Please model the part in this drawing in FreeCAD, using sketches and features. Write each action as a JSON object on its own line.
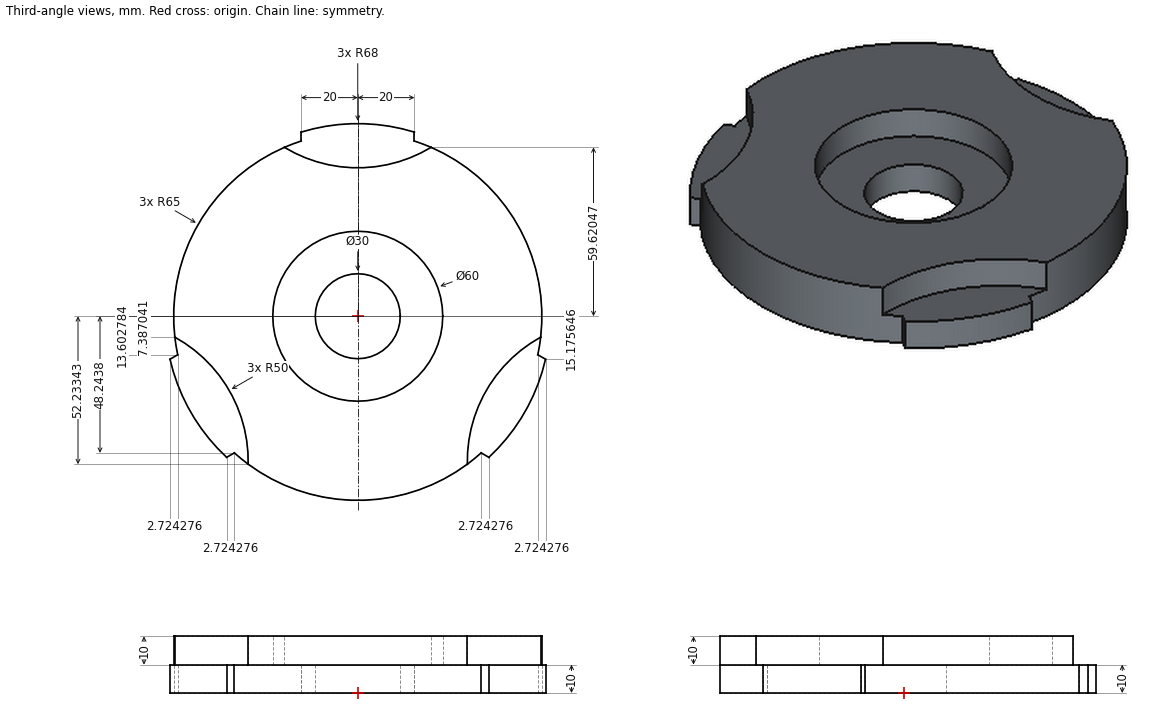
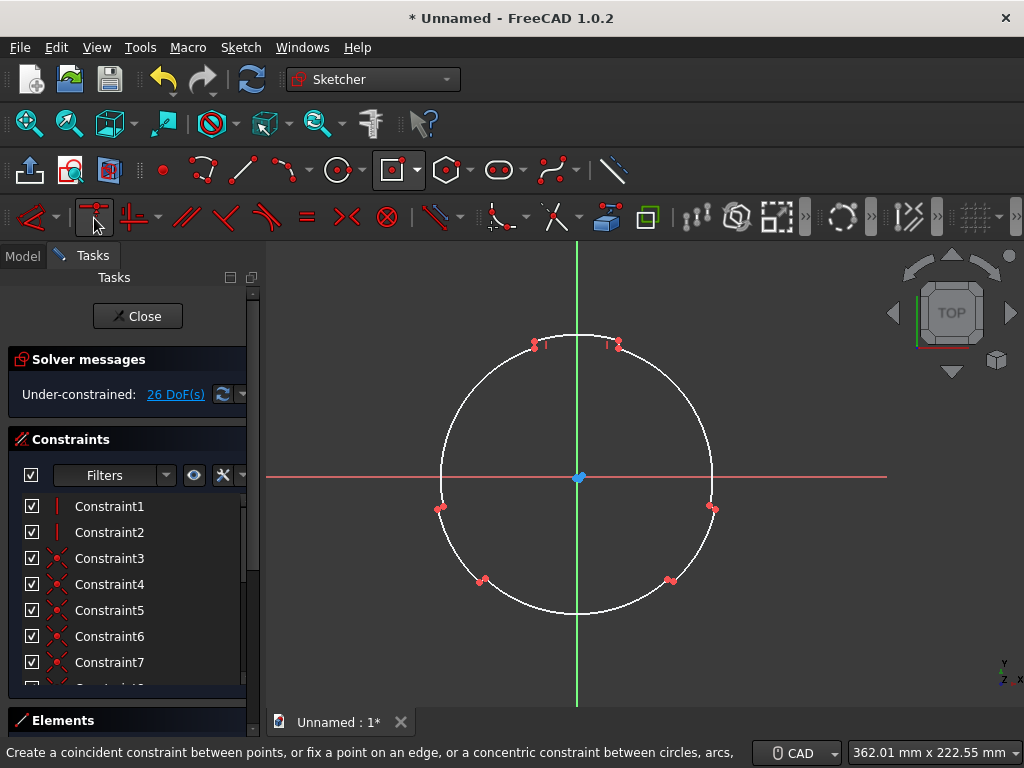
{"action": "left_click", "coordinate": [594, 335]}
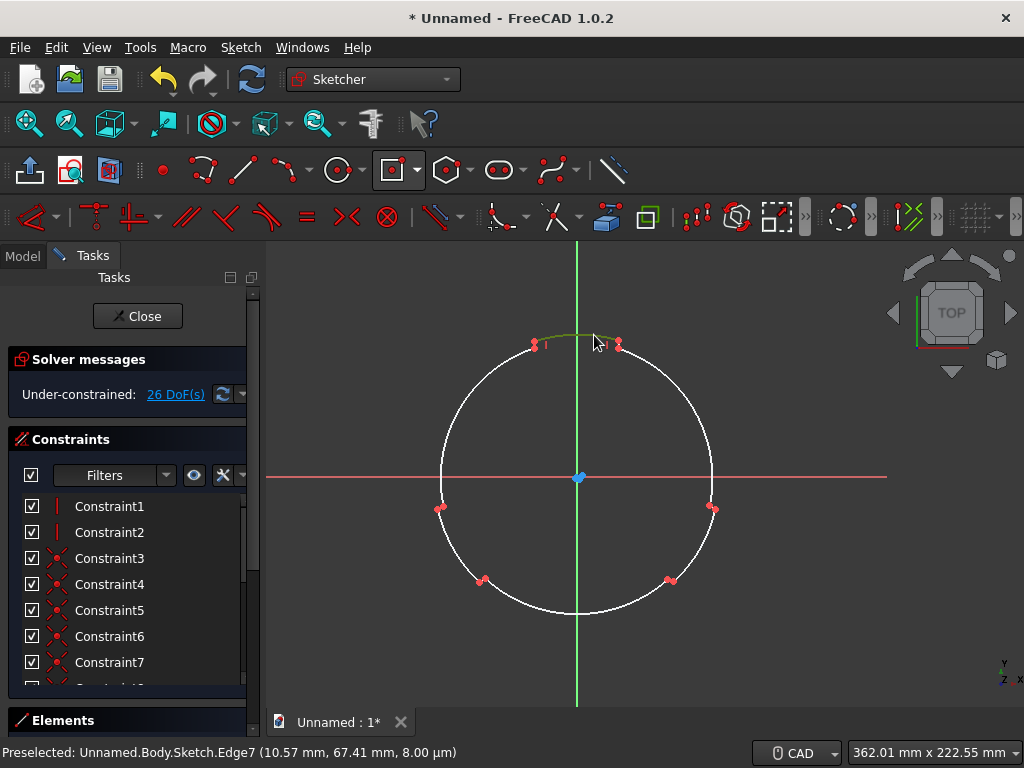
{"action": "left_click", "coordinate": [446, 534]}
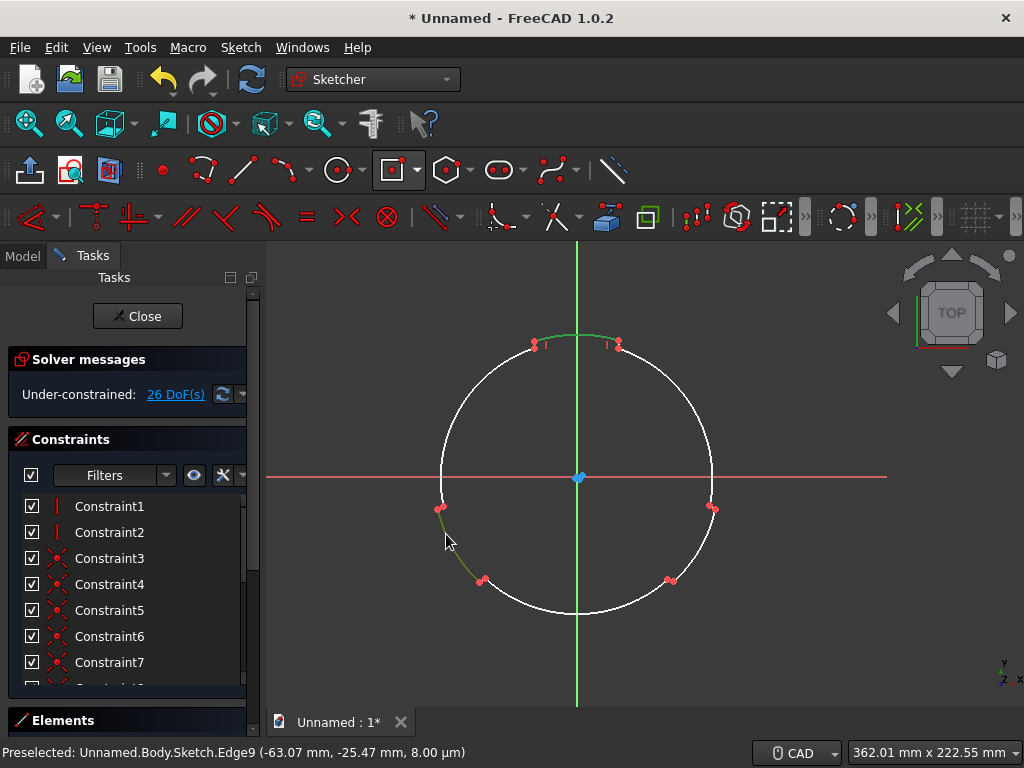
{"action": "left_click", "coordinate": [94, 218]}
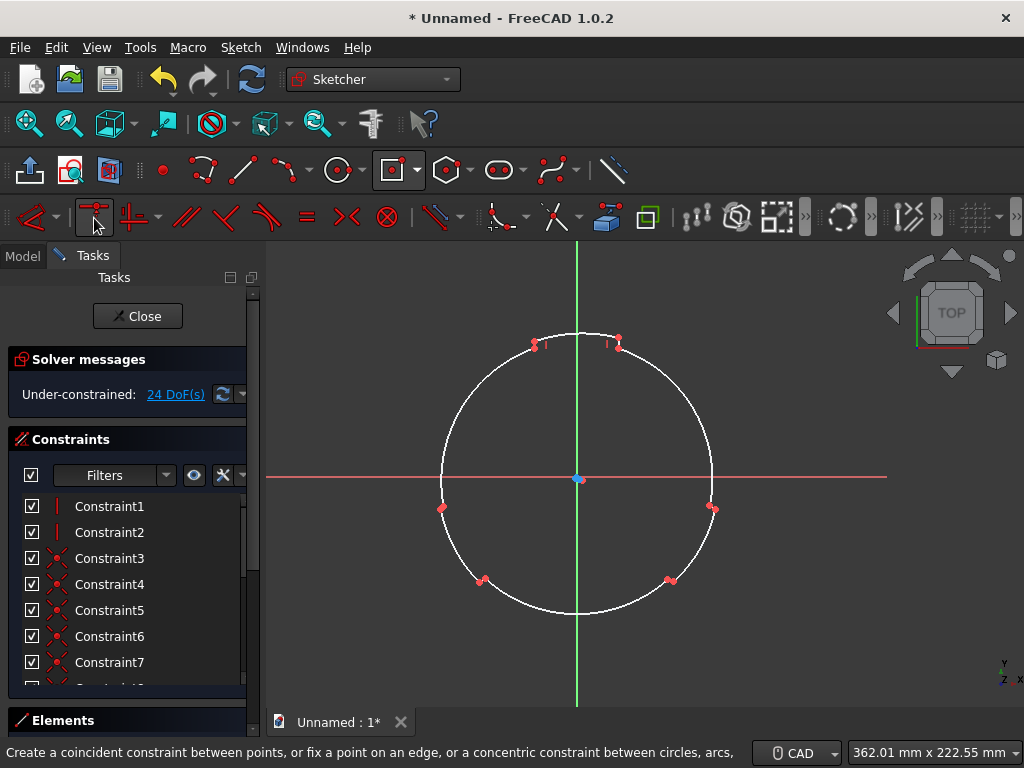
{"action": "left_click", "coordinate": [593, 334]}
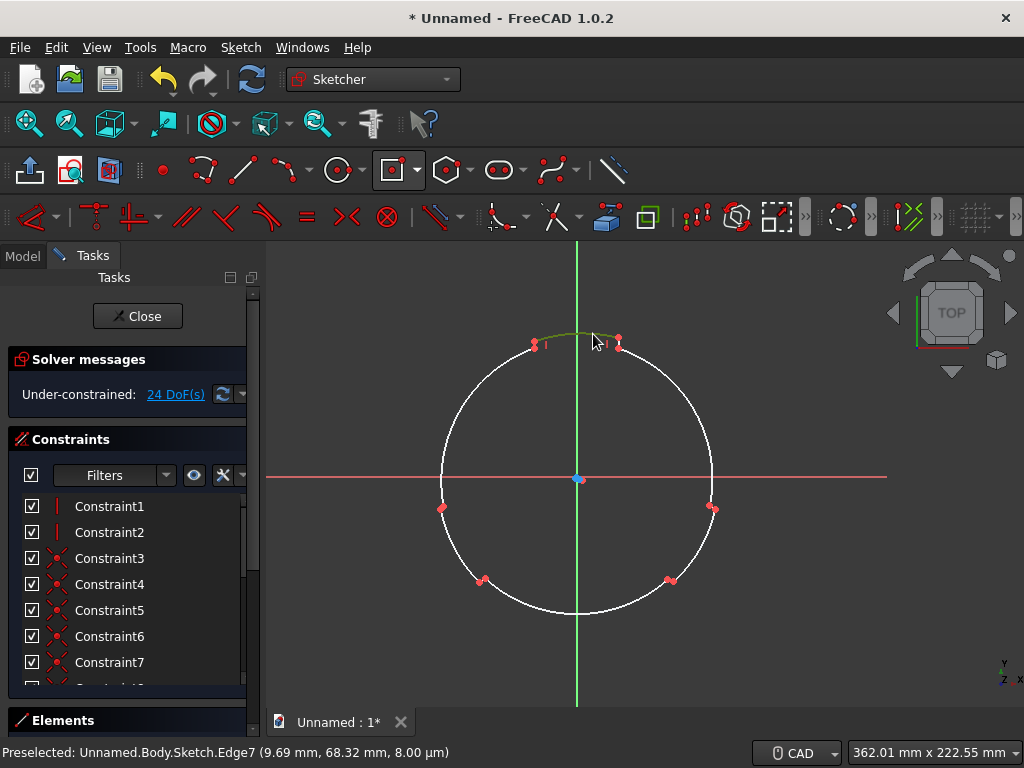
{"action": "left_click", "coordinate": [537, 608]}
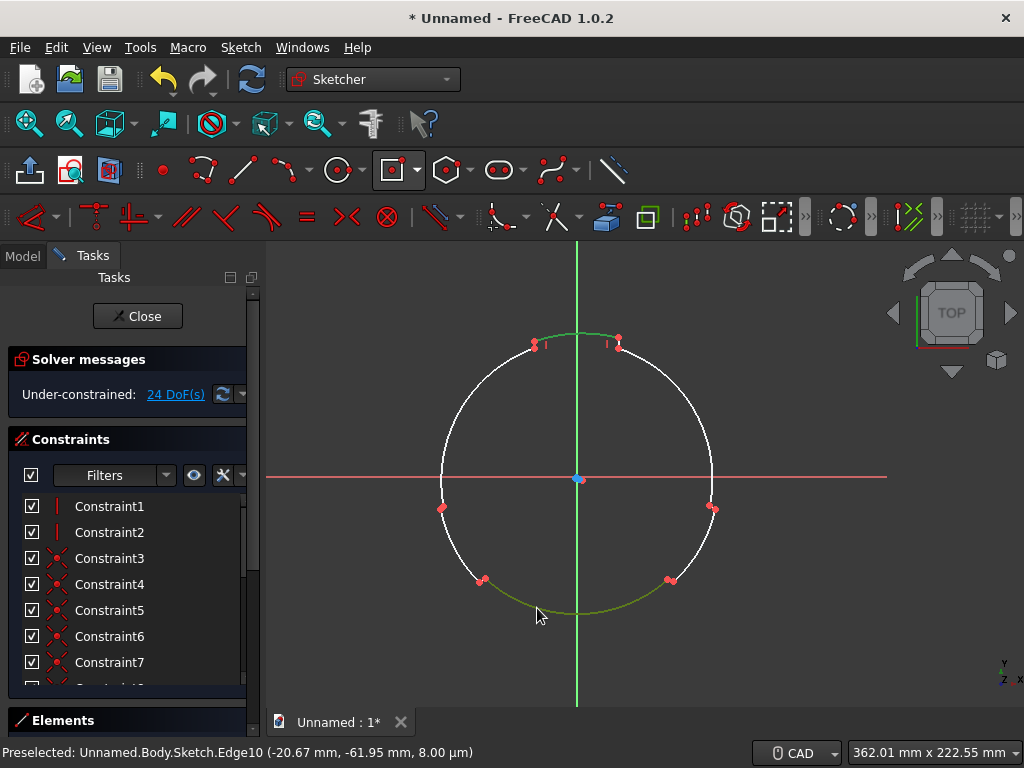
{"action": "left_click", "coordinate": [94, 218]}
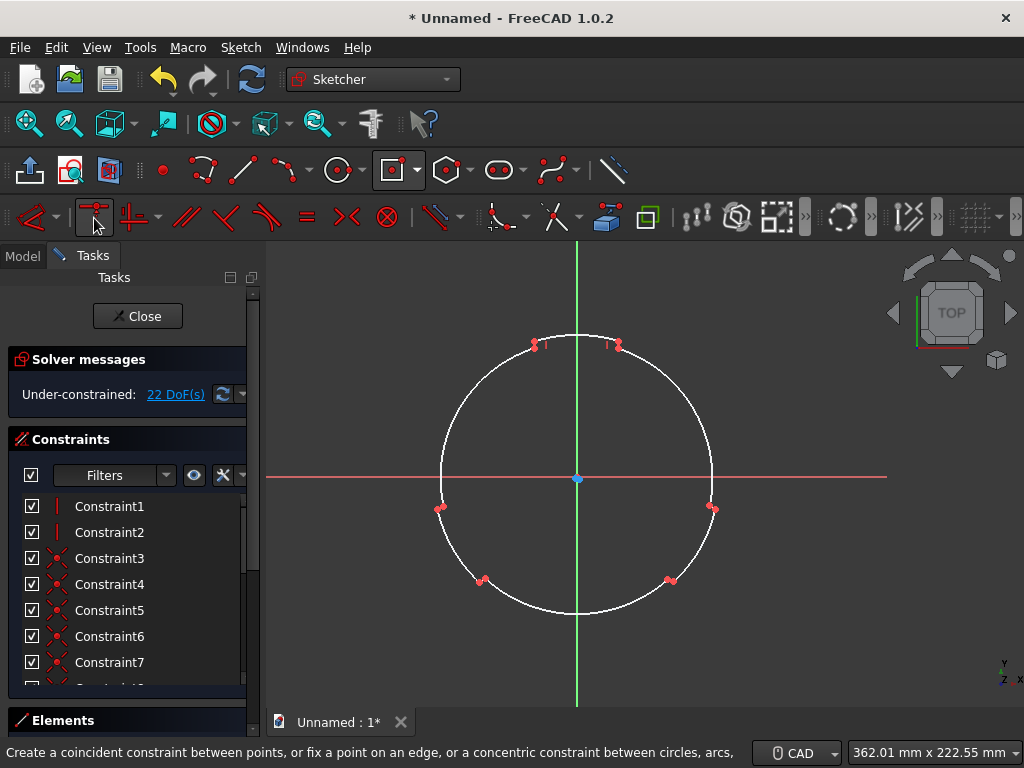
{"action": "left_click", "coordinate": [594, 336]}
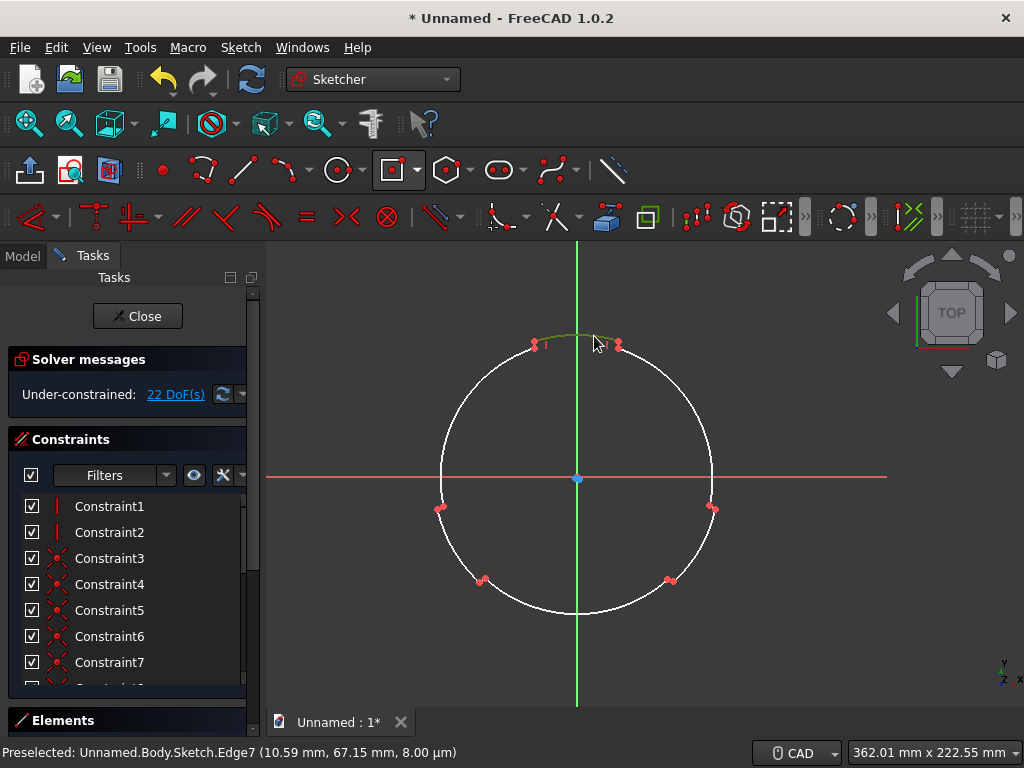
{"action": "left_click", "coordinate": [691, 563]}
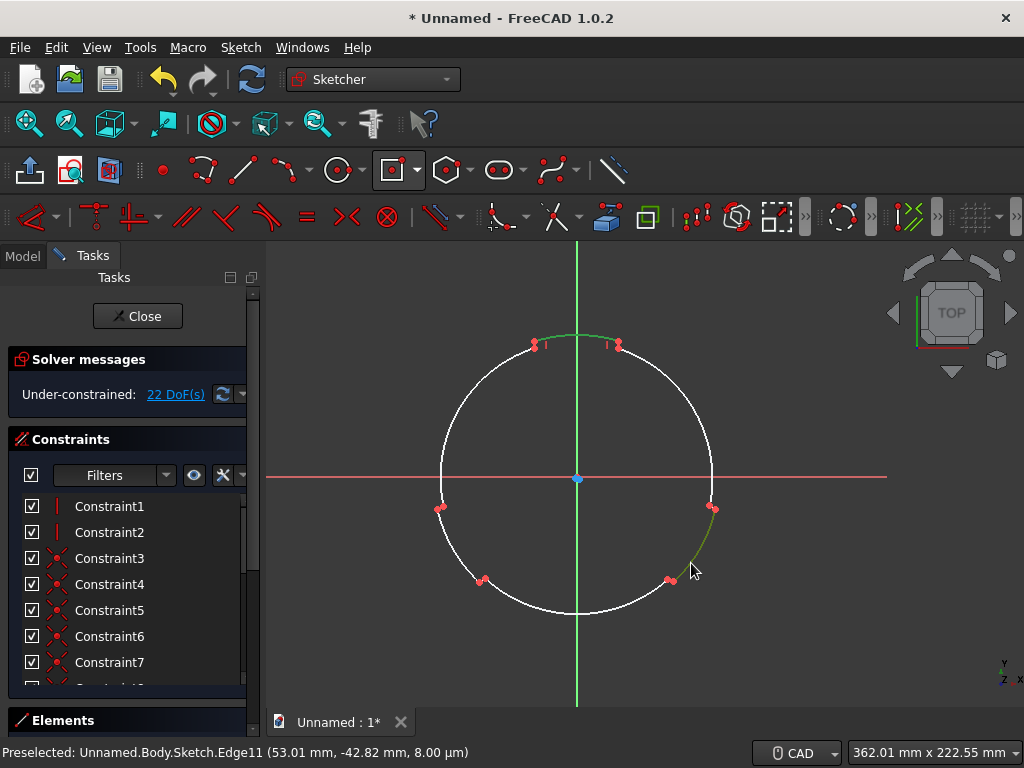
{"action": "key", "text": "c"}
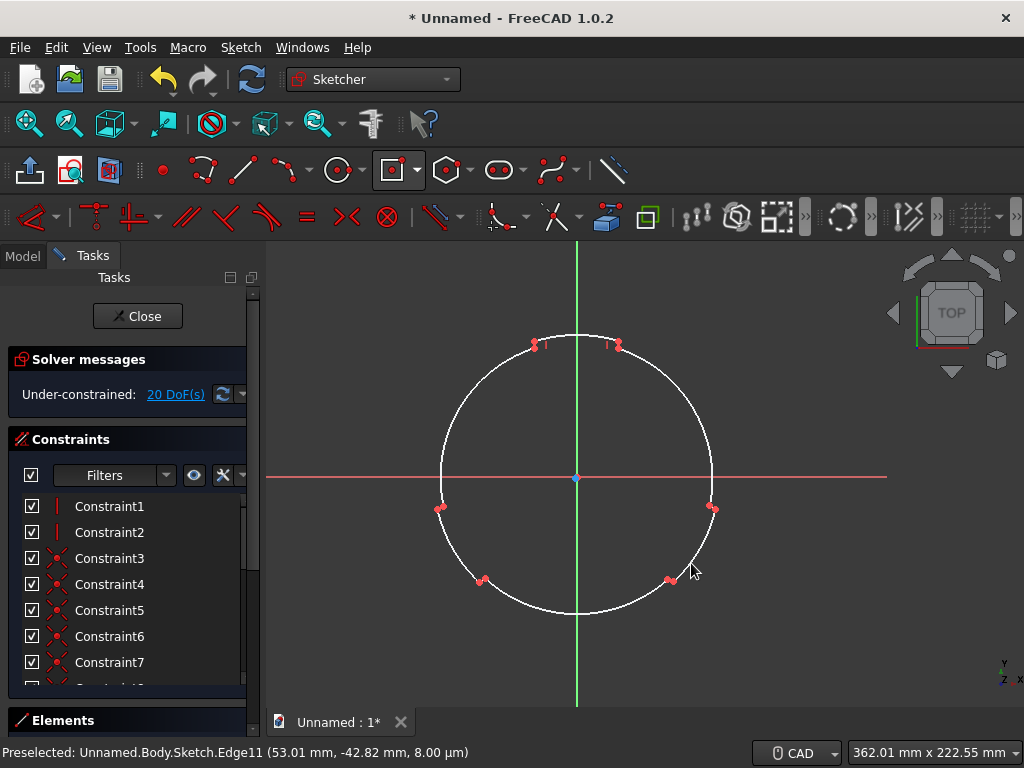
{"action": "left_click", "coordinate": [594, 336]}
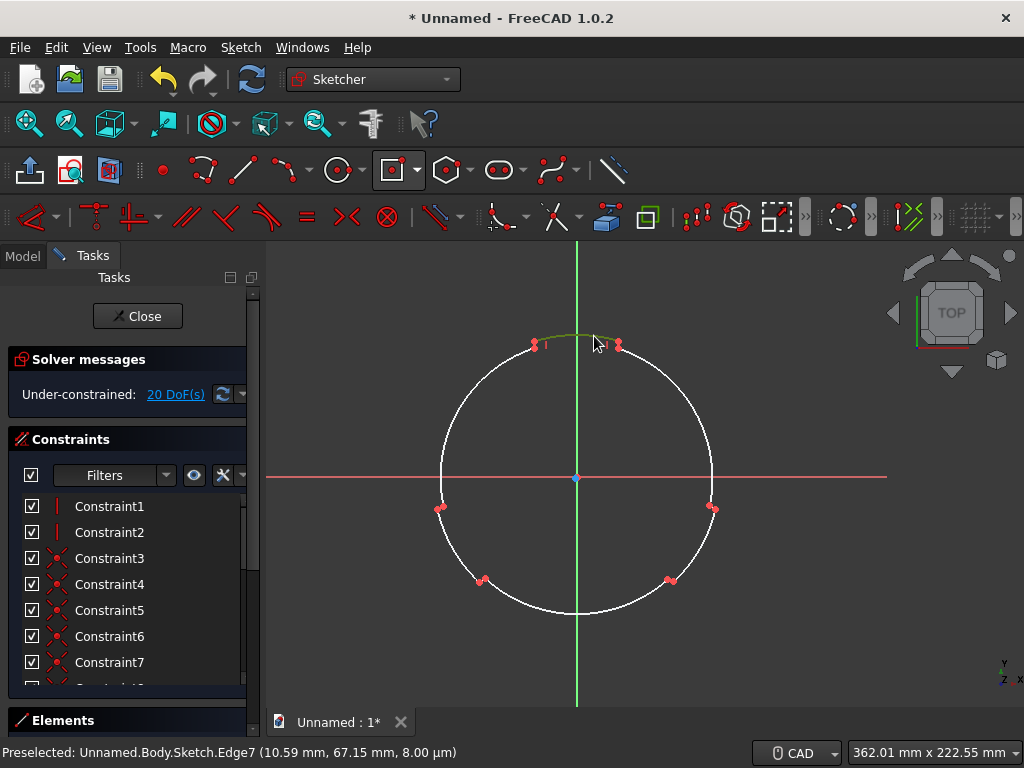
{"action": "left_click", "coordinate": [709, 447]}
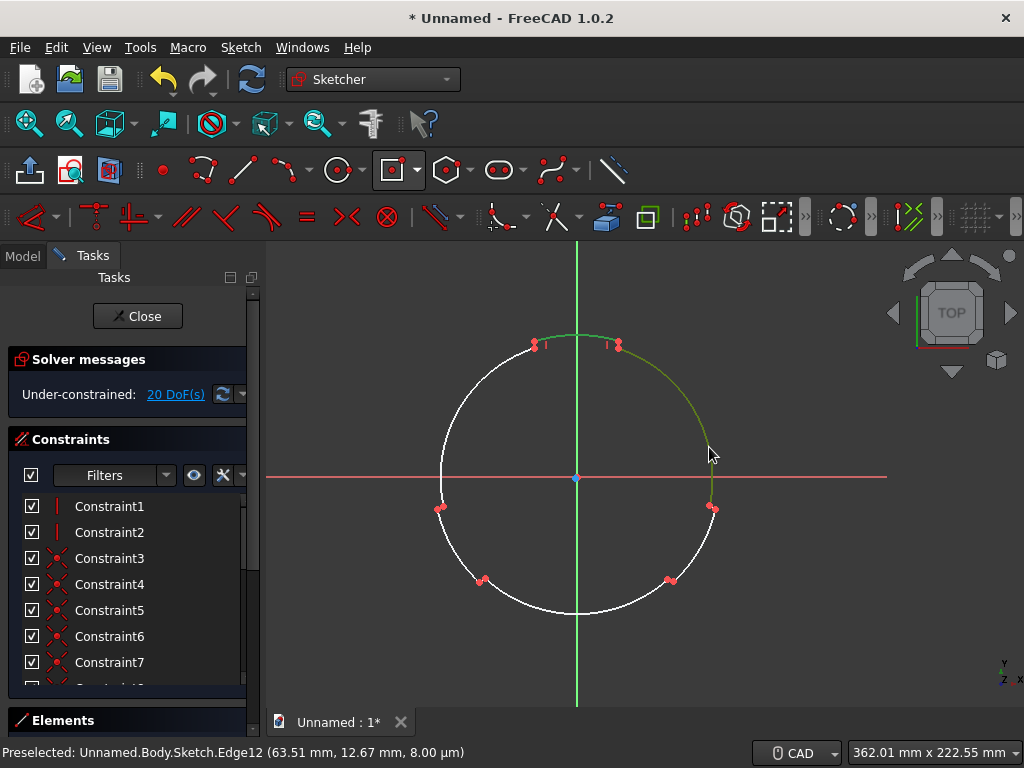
{"action": "key", "text": "c"}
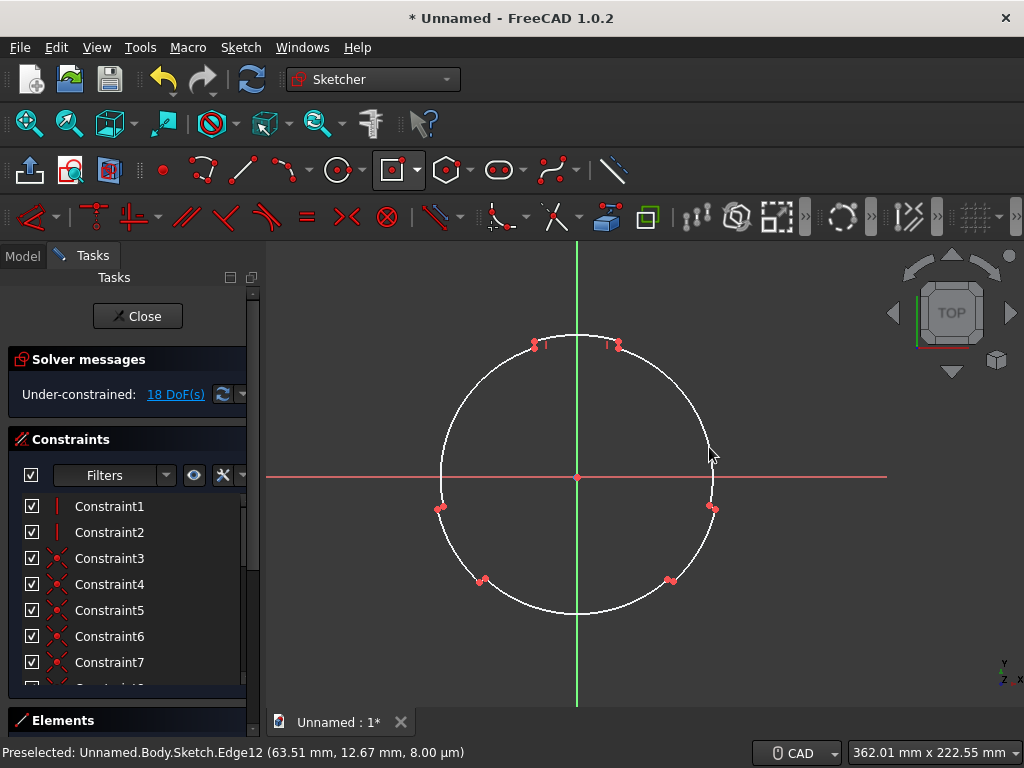
{"action": "left_click_drag", "start_coordinate": [567, 467], "coordinate": [587, 488]}